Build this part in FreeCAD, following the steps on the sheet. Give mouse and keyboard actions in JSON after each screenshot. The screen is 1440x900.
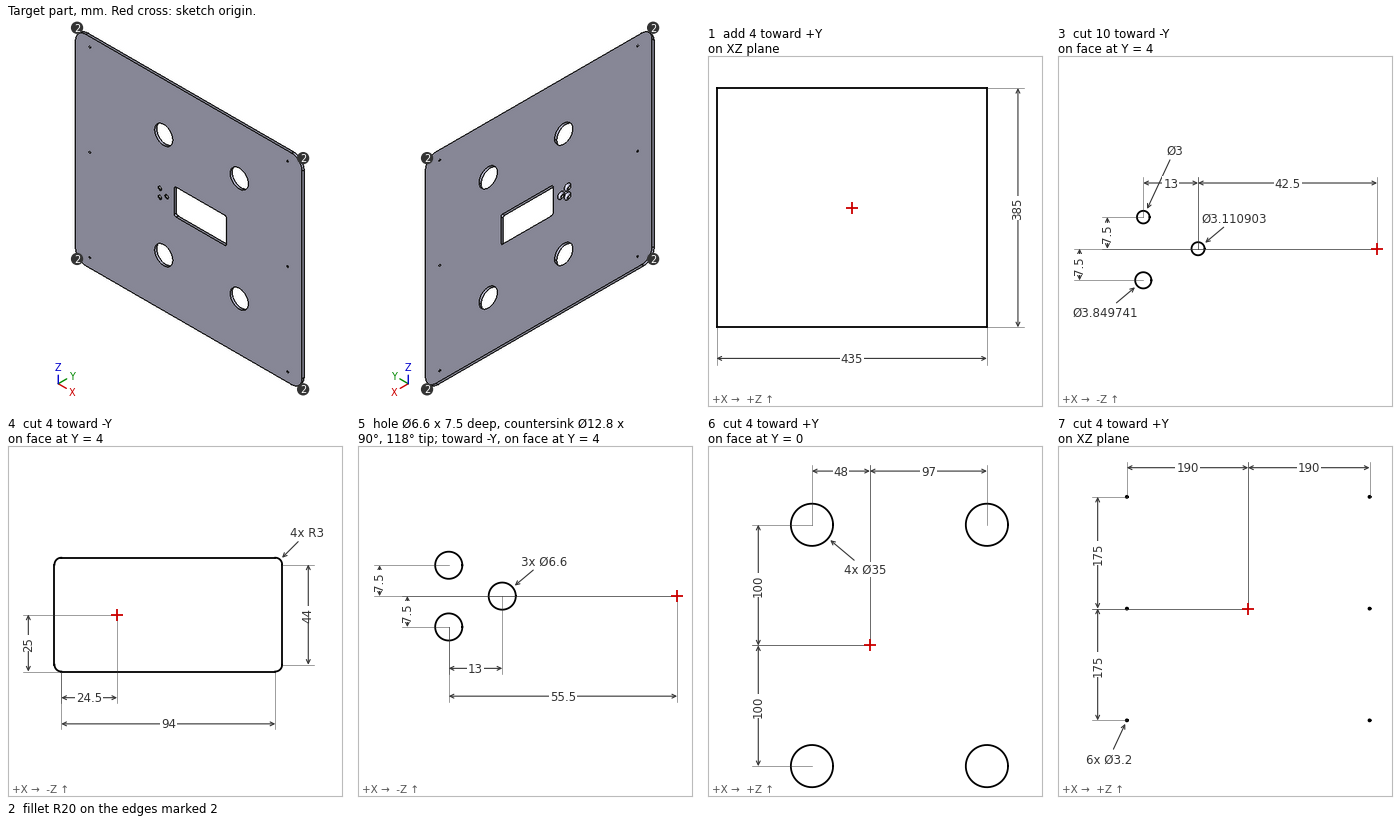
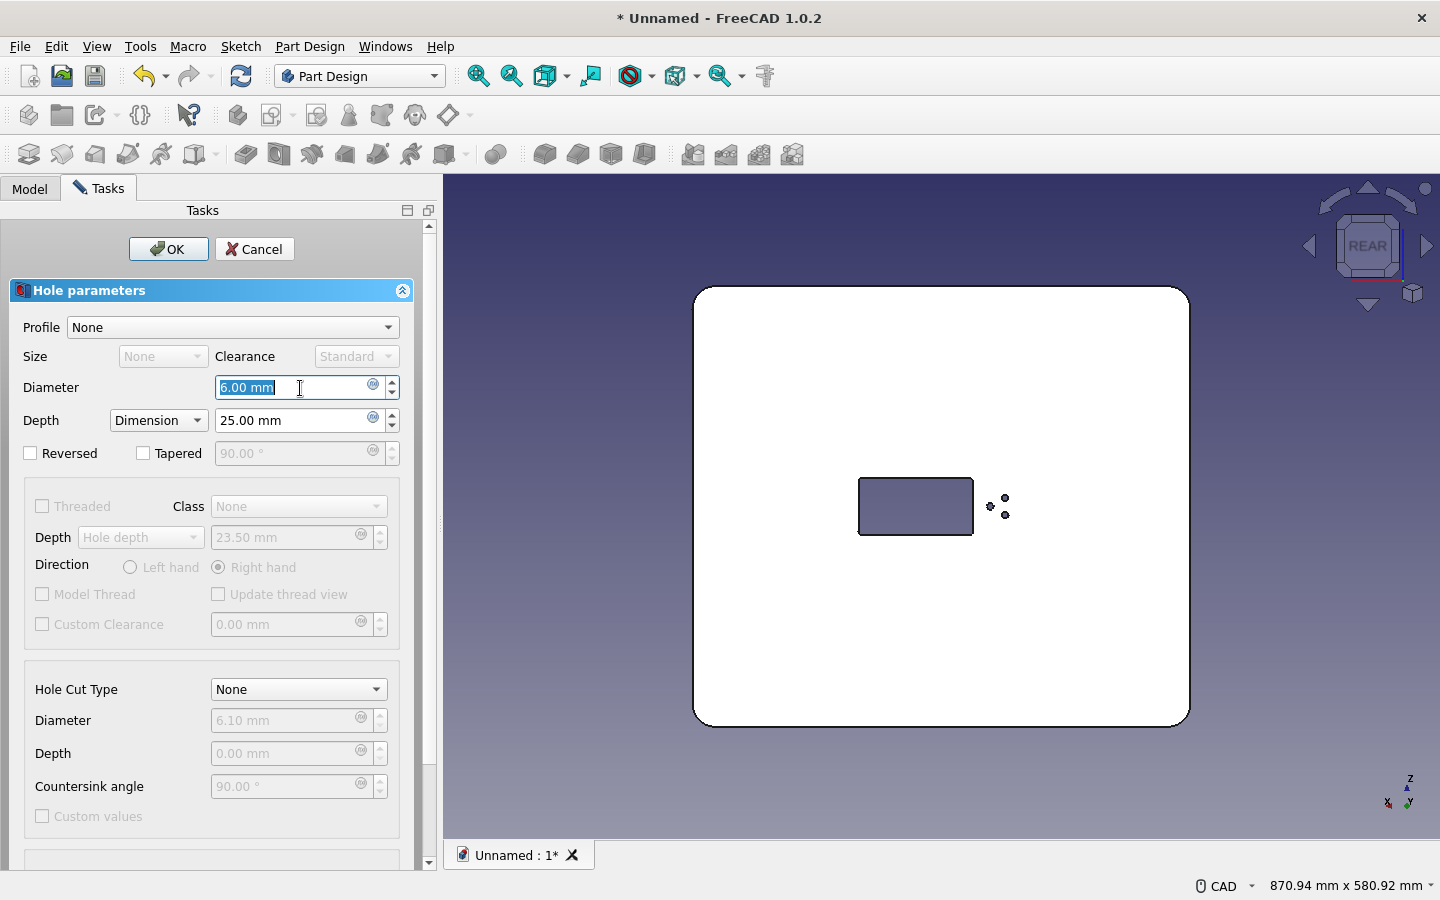
{"action": "type", "text": "6.6"}
{"action": "key", "text": "Tab"}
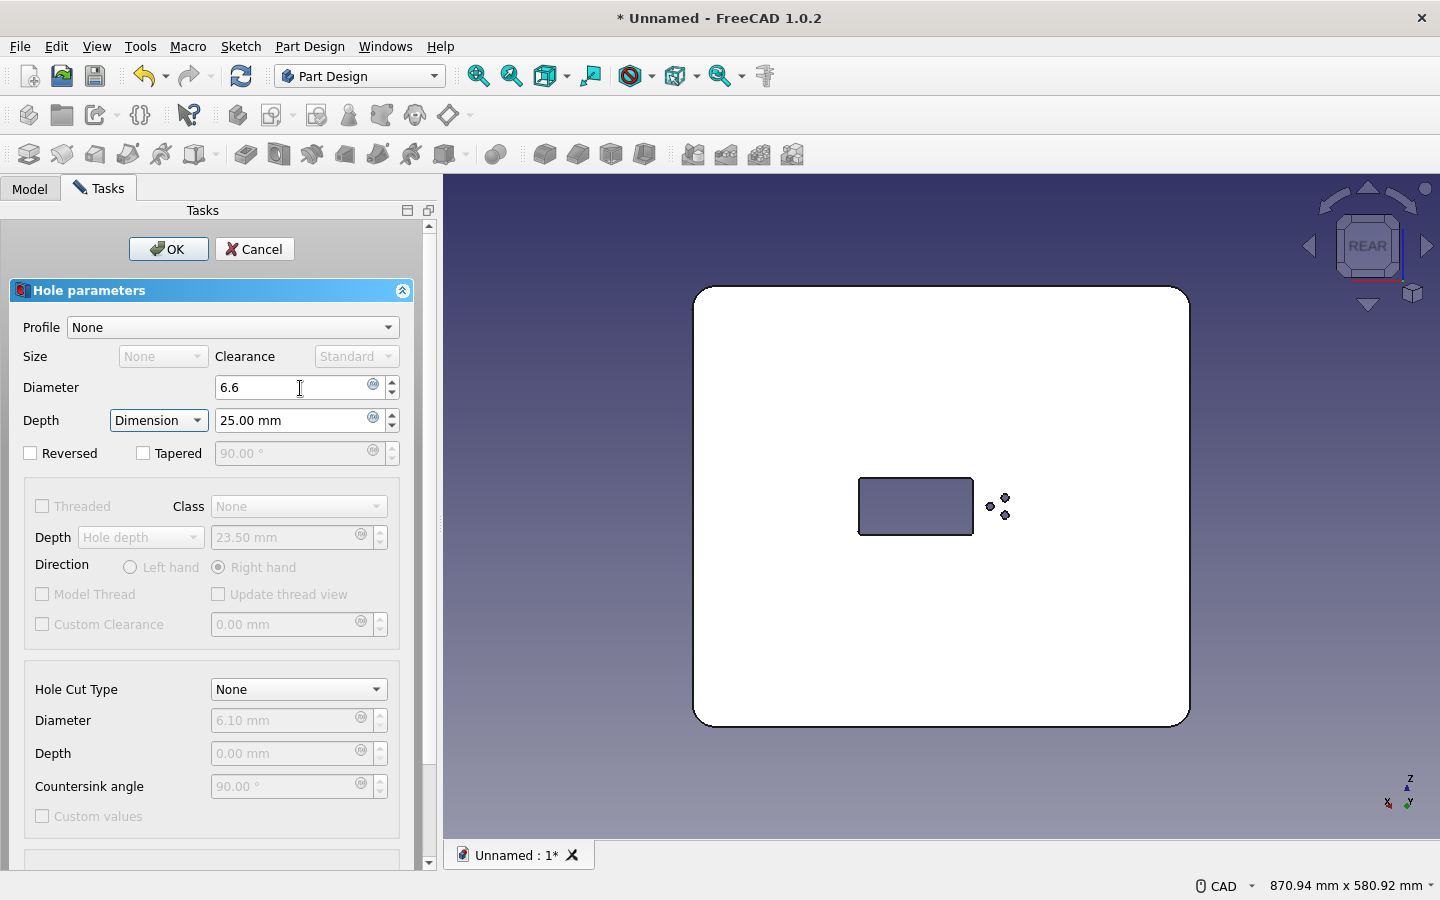
{"action": "triple_click", "coordinate": [300, 420]}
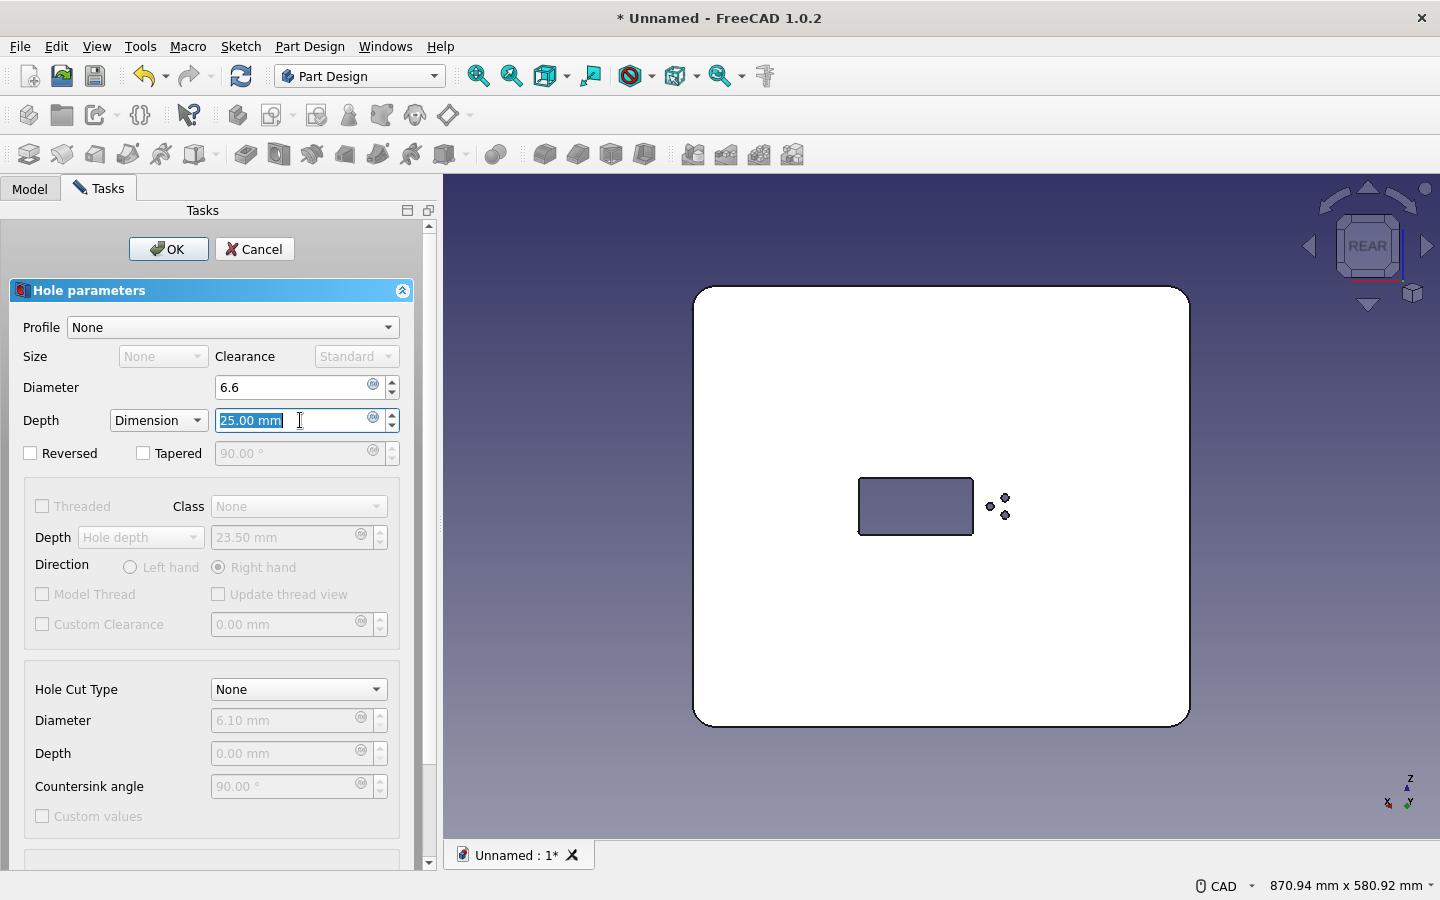
{"action": "type", "text": "7.5"}
{"action": "key", "text": "Tab"}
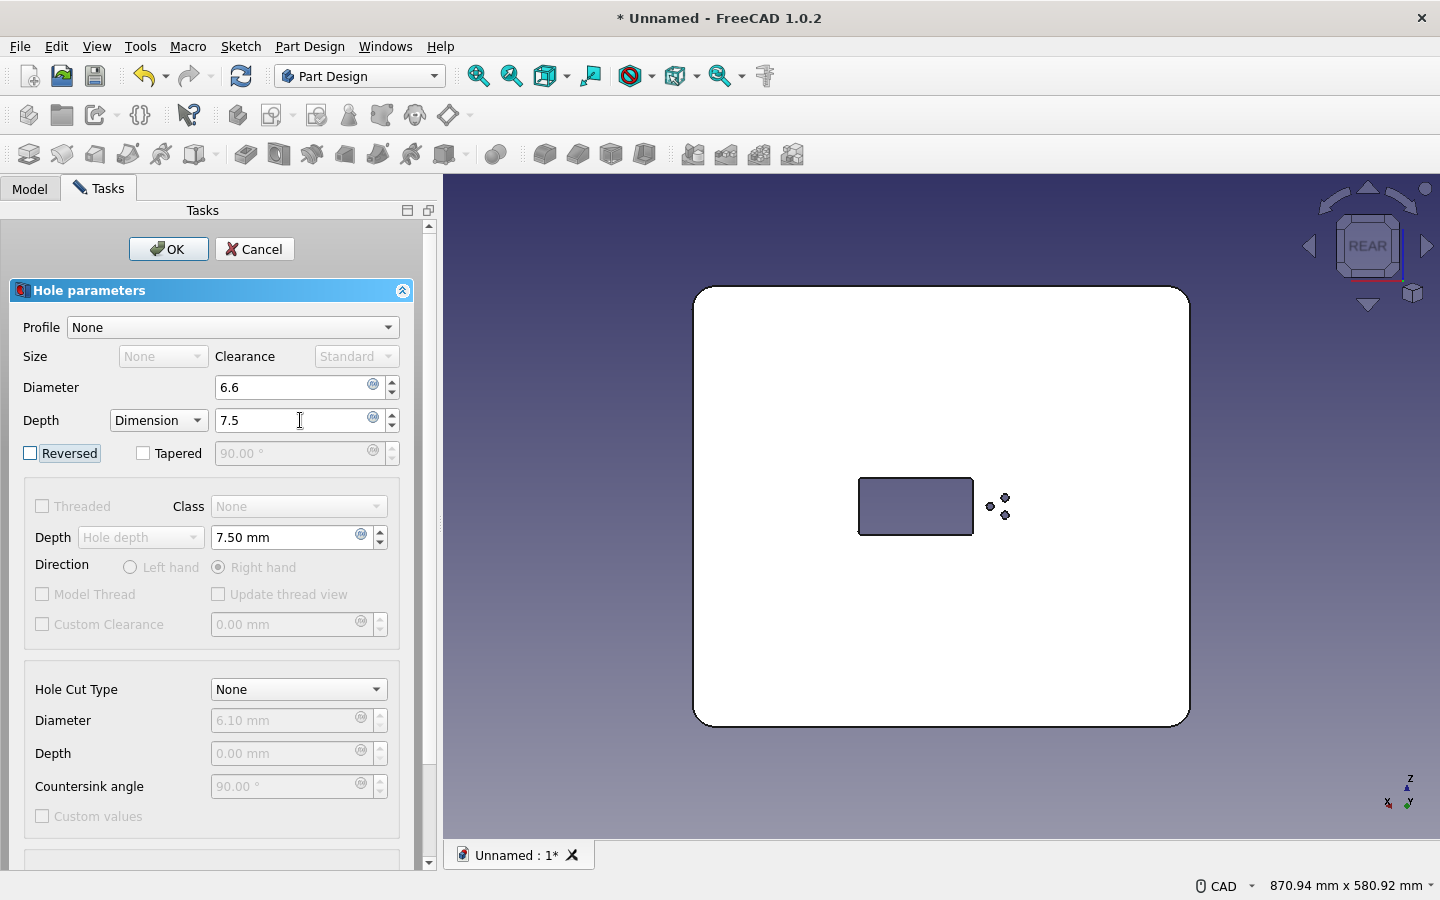
{"action": "left_click", "coordinate": [300, 690]}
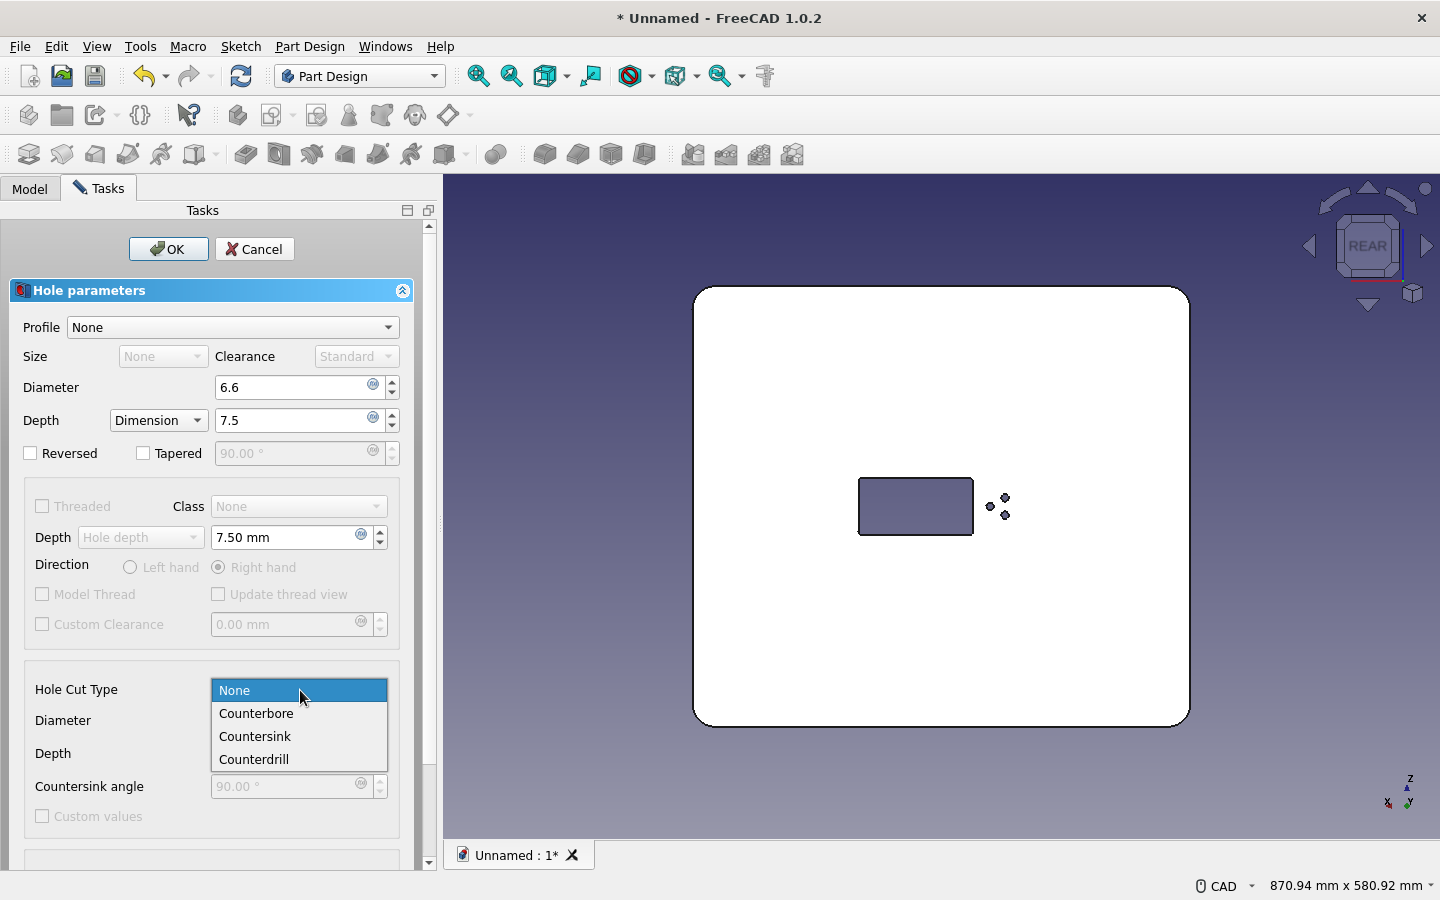
{"action": "left_click", "coordinate": [298, 736]}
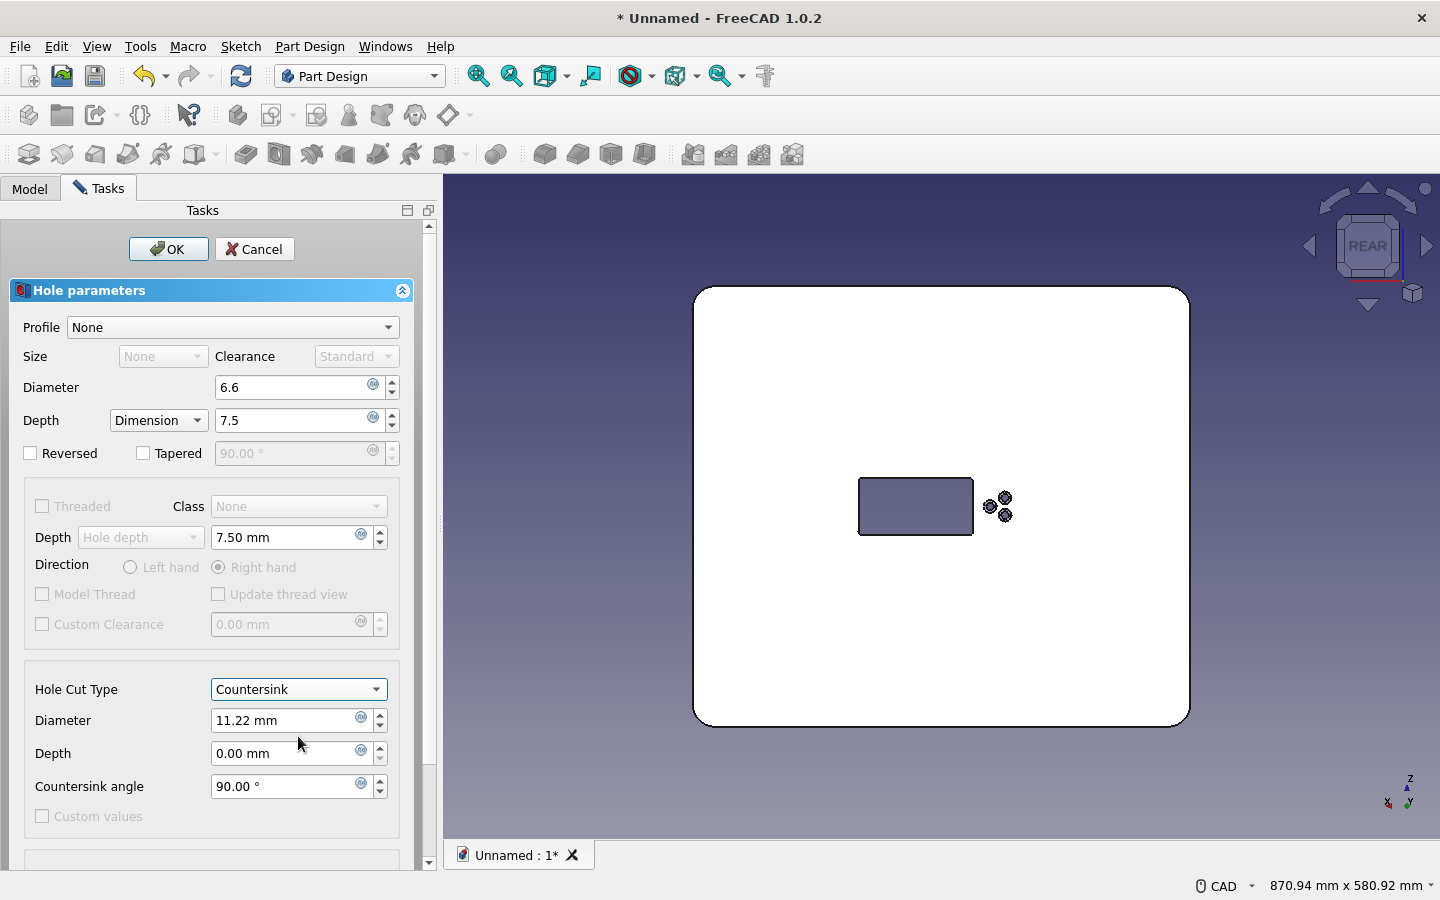
{"action": "triple_click", "coordinate": [292, 720]}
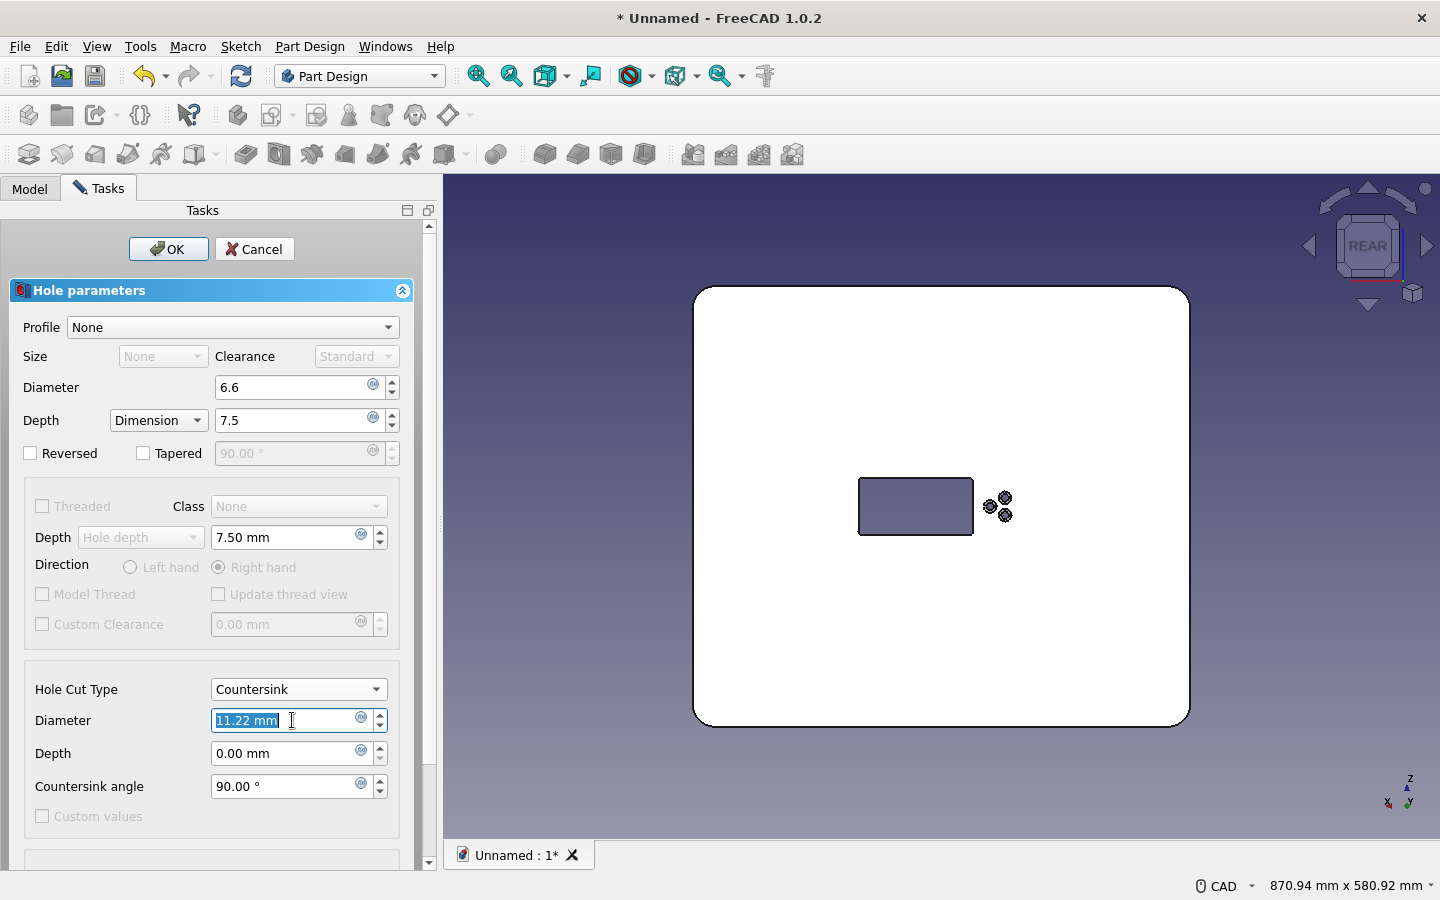
{"action": "type", "text": "12.8"}
{"action": "key", "text": "Tab"}